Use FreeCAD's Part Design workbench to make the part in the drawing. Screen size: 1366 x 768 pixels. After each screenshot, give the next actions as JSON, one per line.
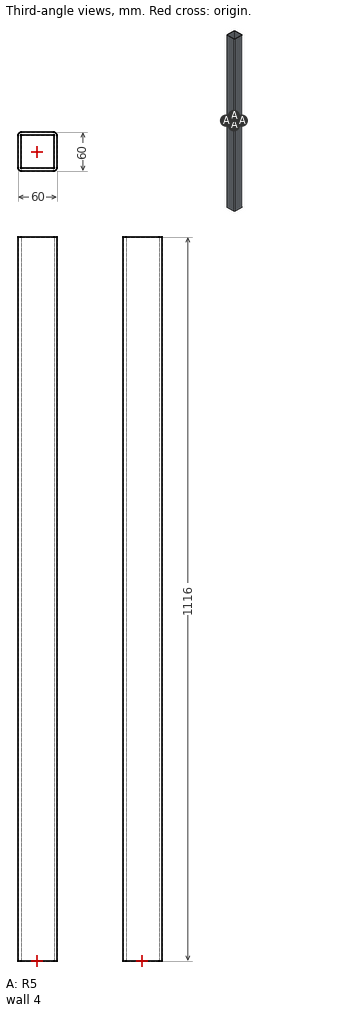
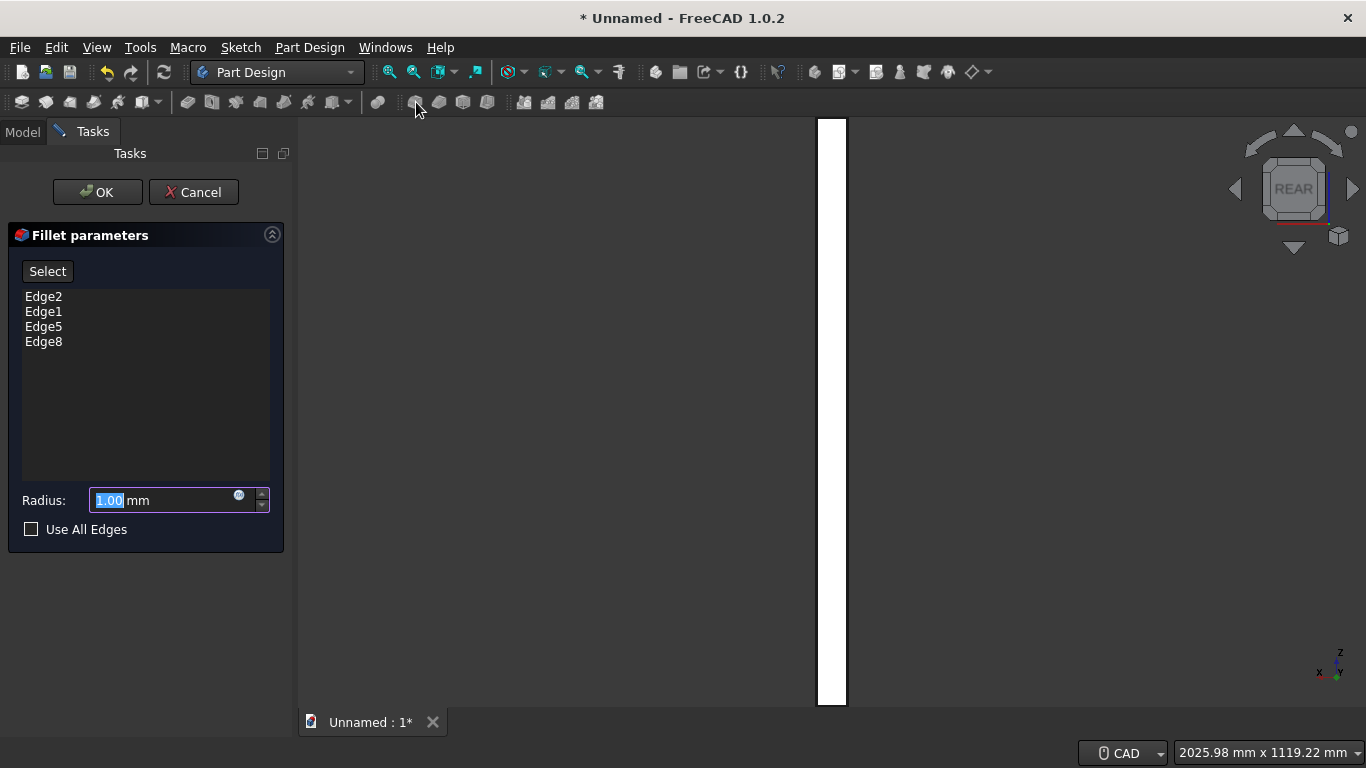
{"action": "type", "text": "5"}
{"action": "key", "text": "Tab"}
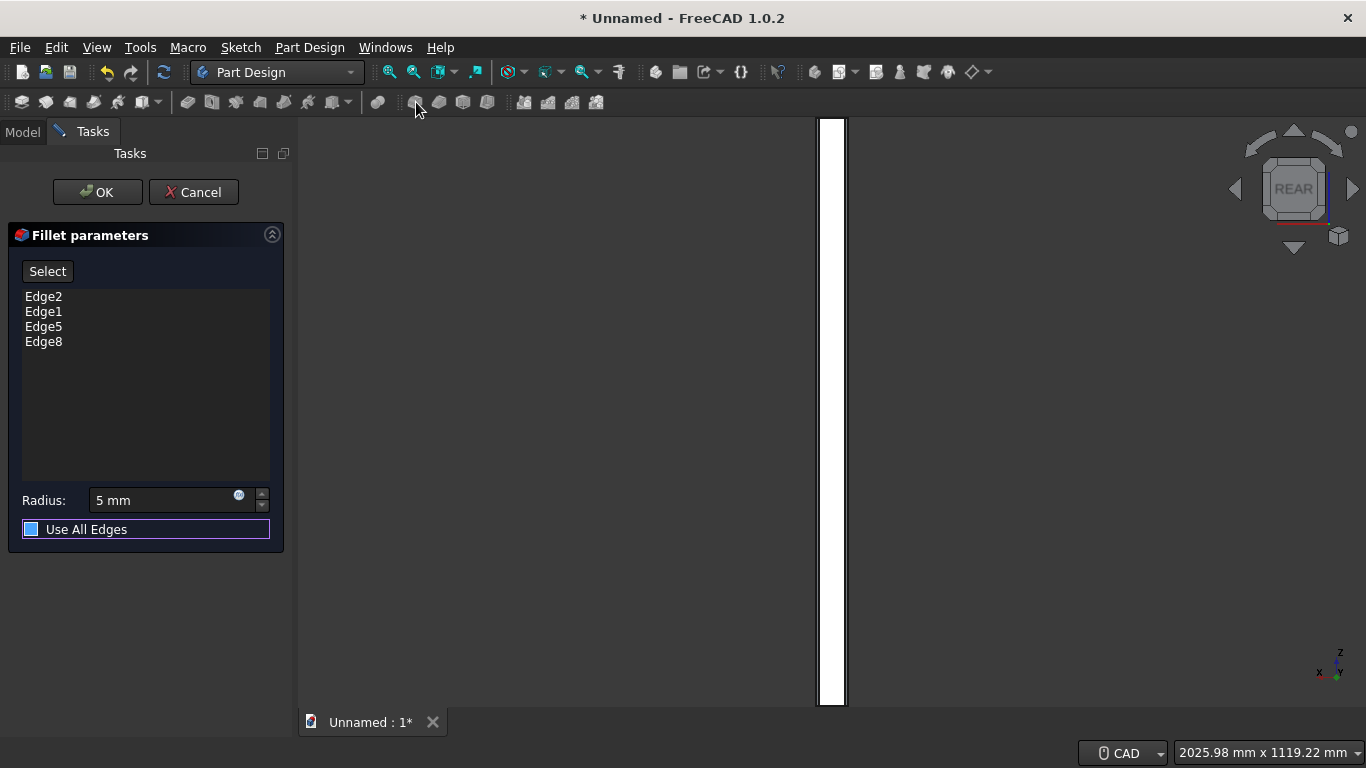
{"action": "left_click", "coordinate": [98, 192]}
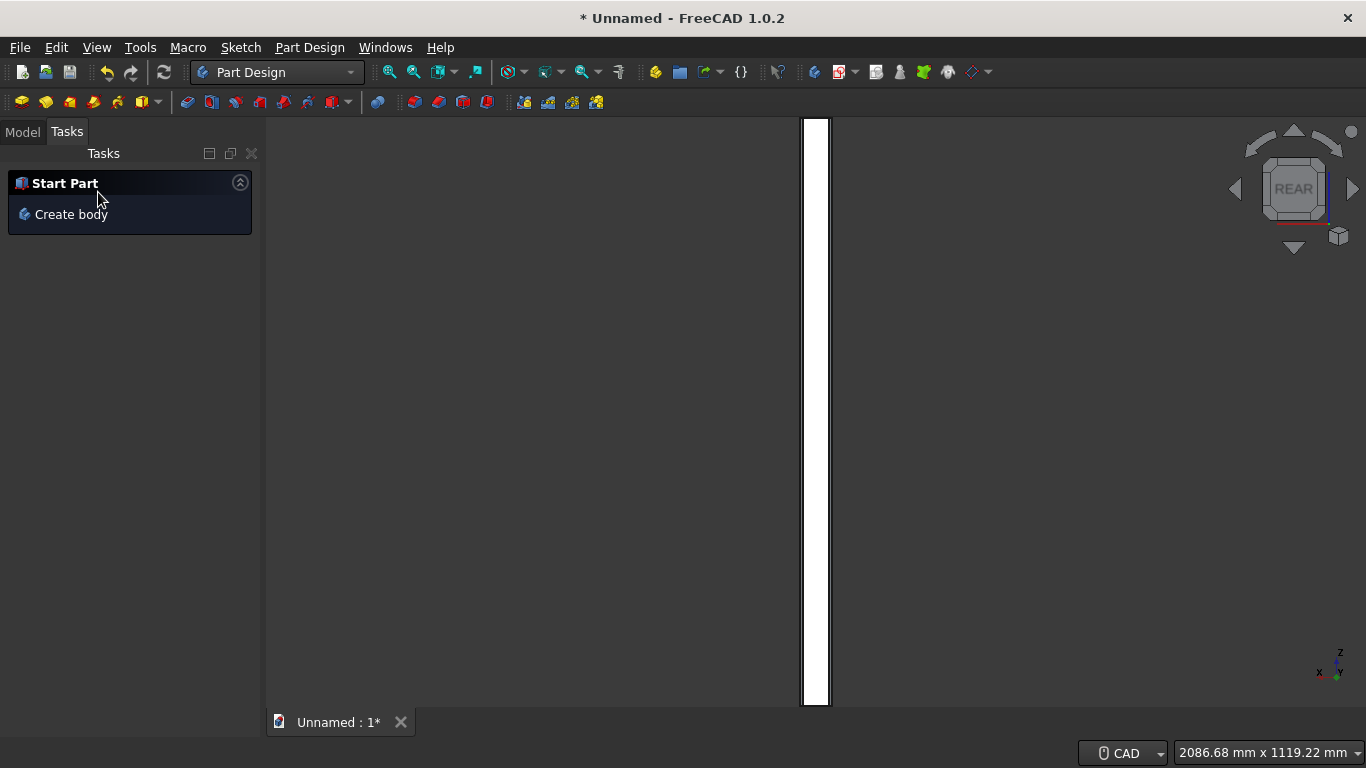
{"action": "key", "text": "0"}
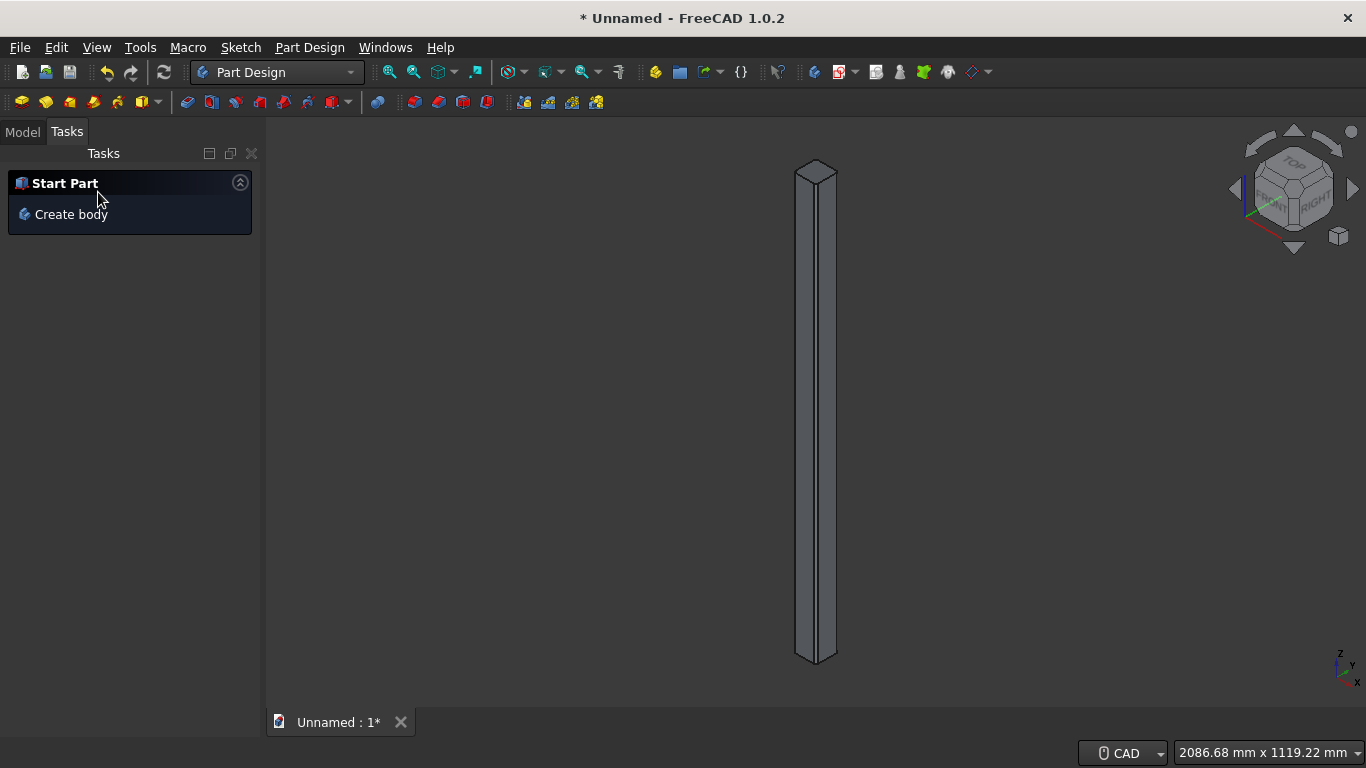
{"action": "left_click", "coordinate": [816, 171]}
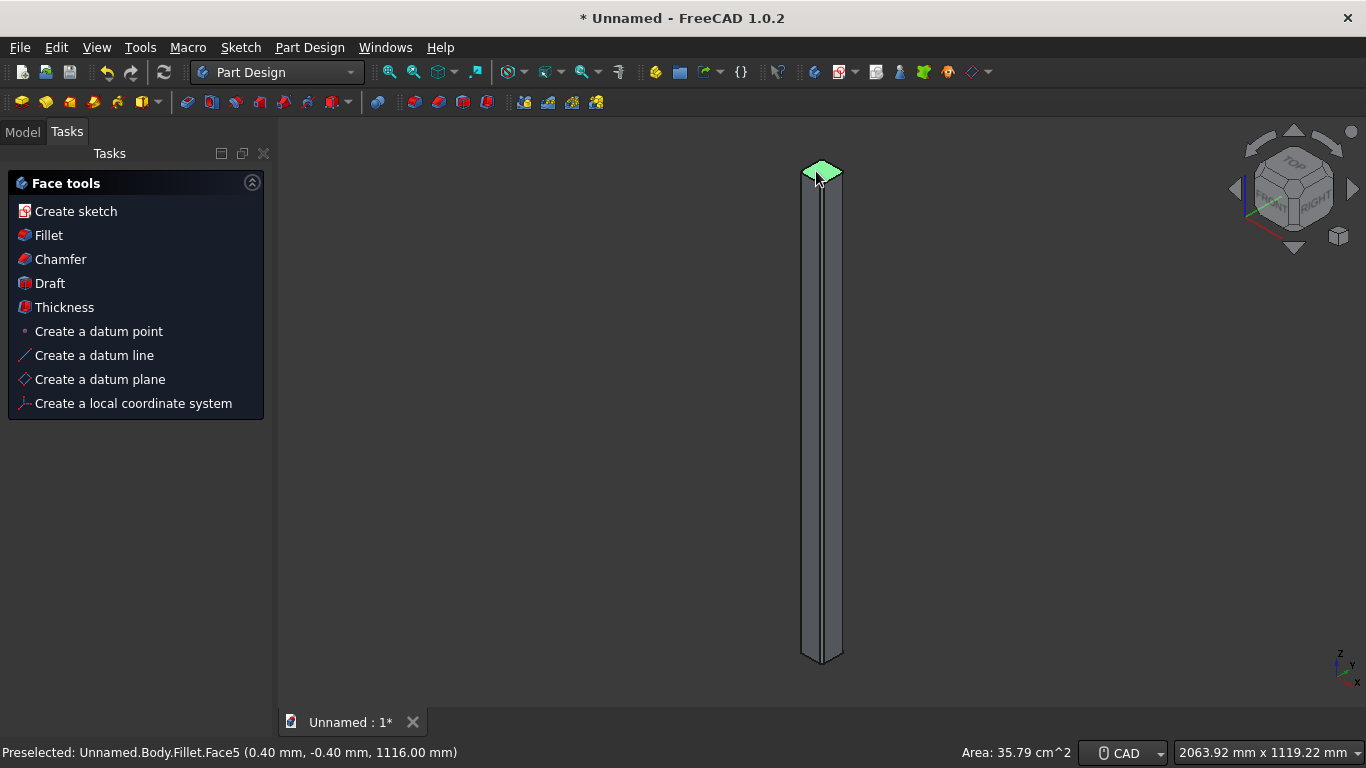
{"action": "key", "text": "2"}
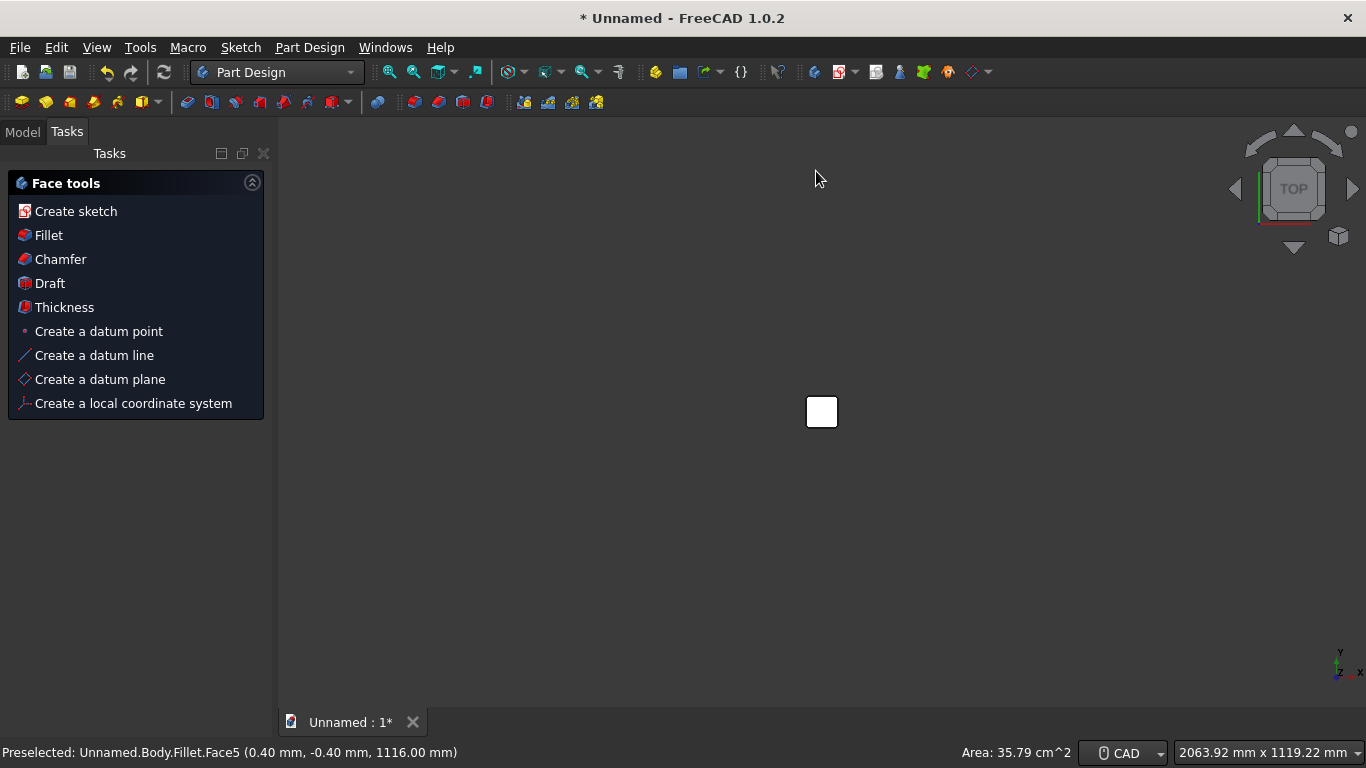
{"action": "left_click", "coordinate": [390, 72]}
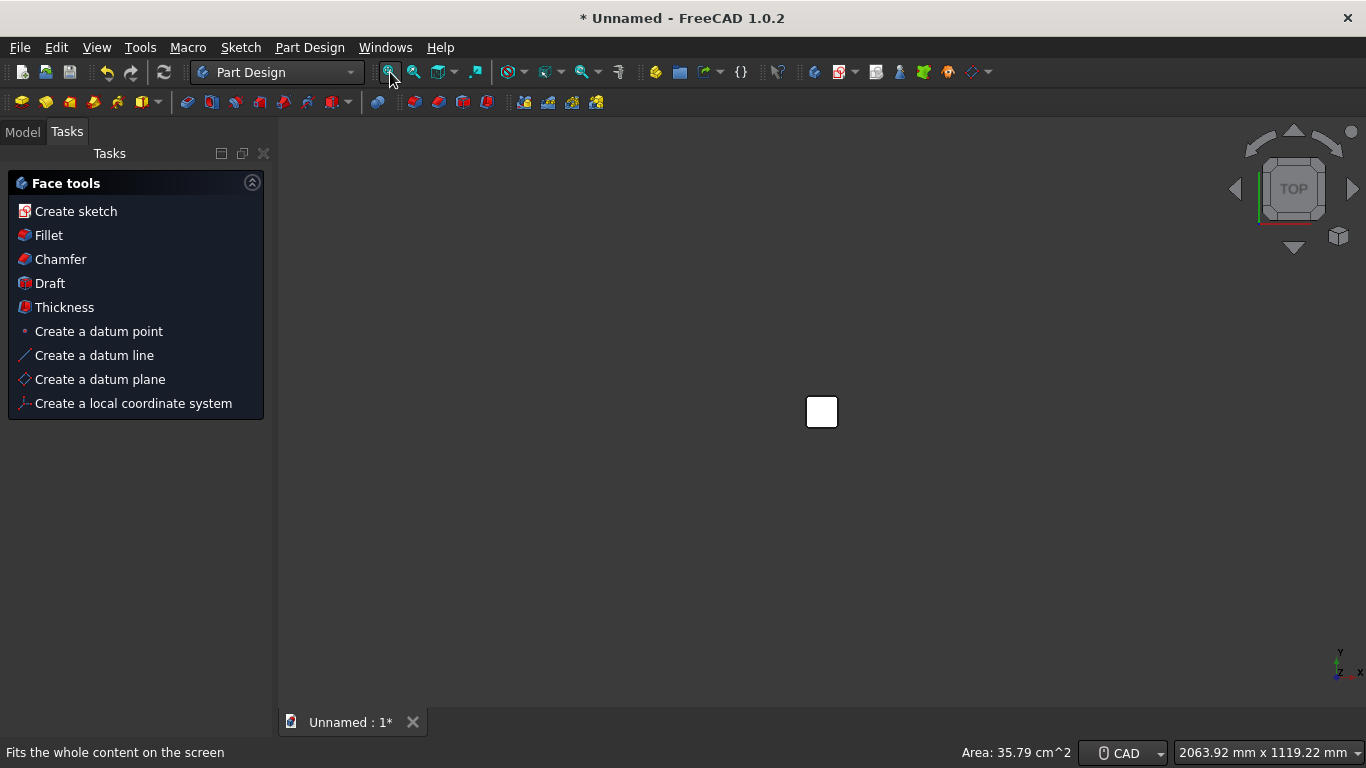
{"action": "key", "text": "1"}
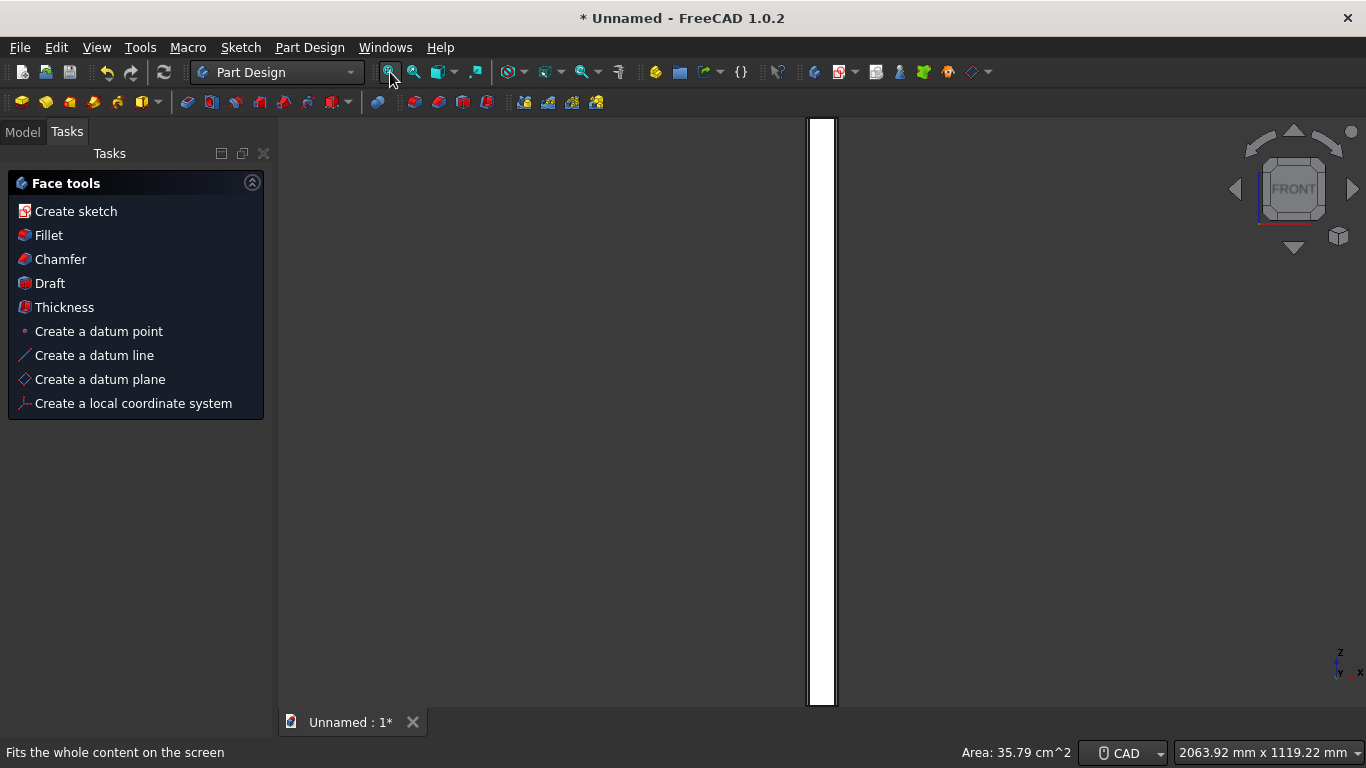
{"action": "key", "text": "3"}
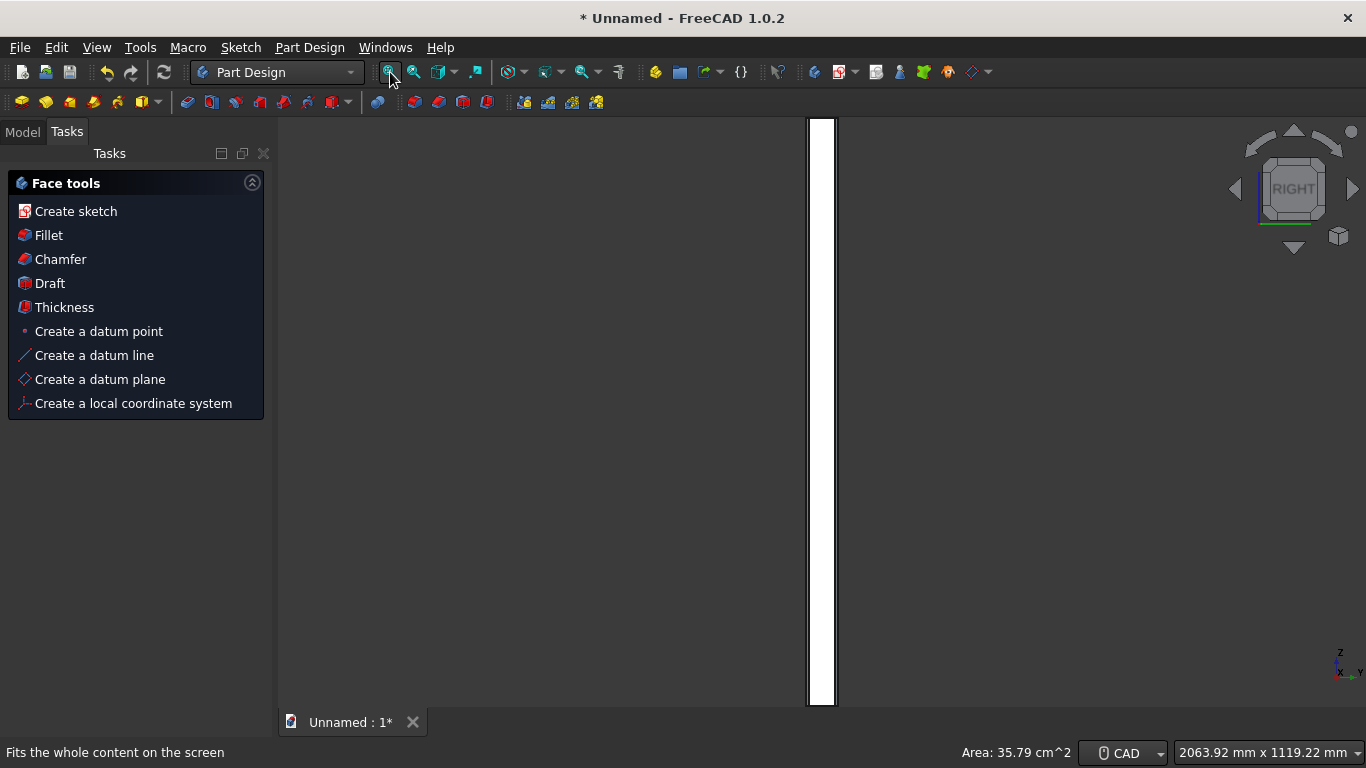
{"action": "key", "text": "5"}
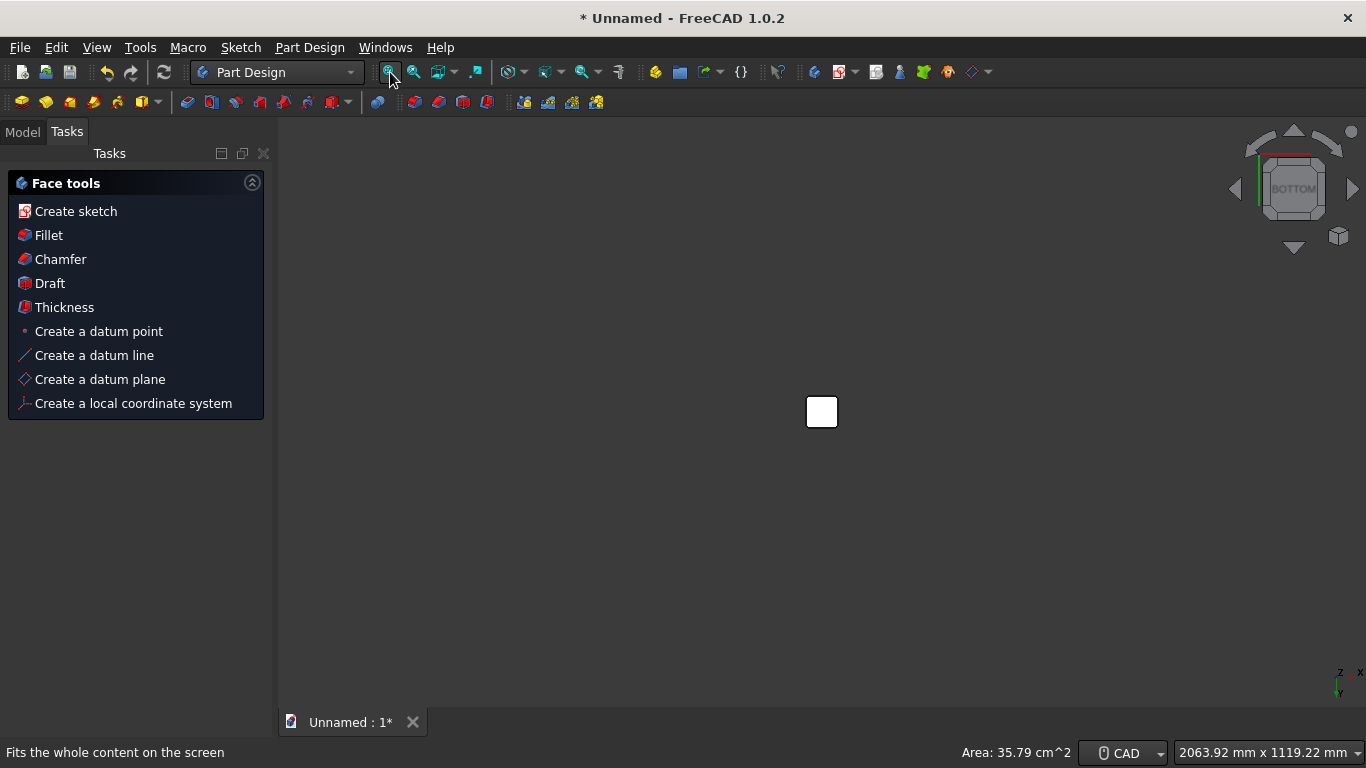
{"action": "left_click", "coordinate": [390, 72]}